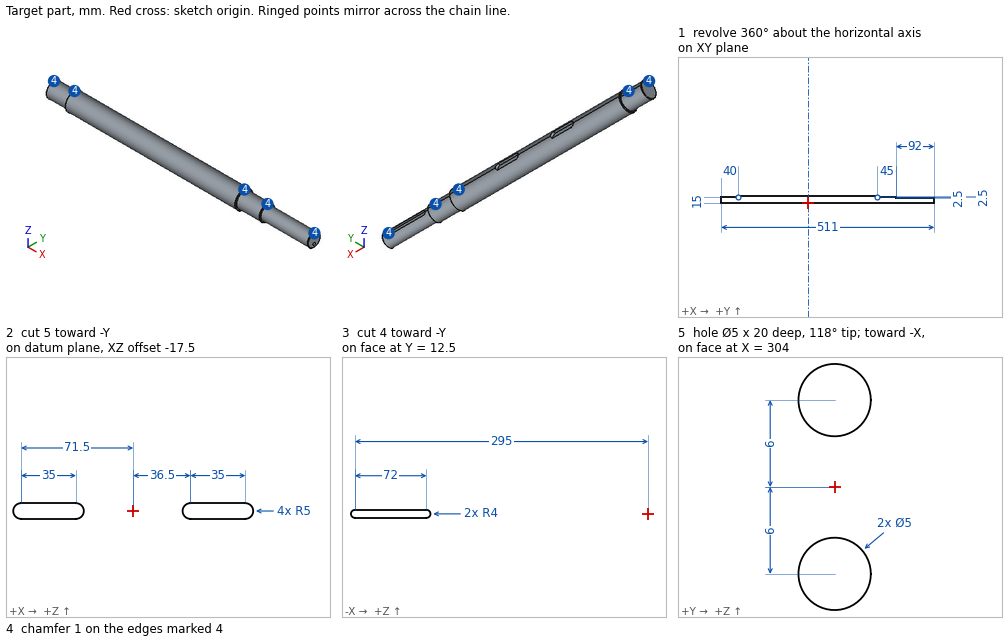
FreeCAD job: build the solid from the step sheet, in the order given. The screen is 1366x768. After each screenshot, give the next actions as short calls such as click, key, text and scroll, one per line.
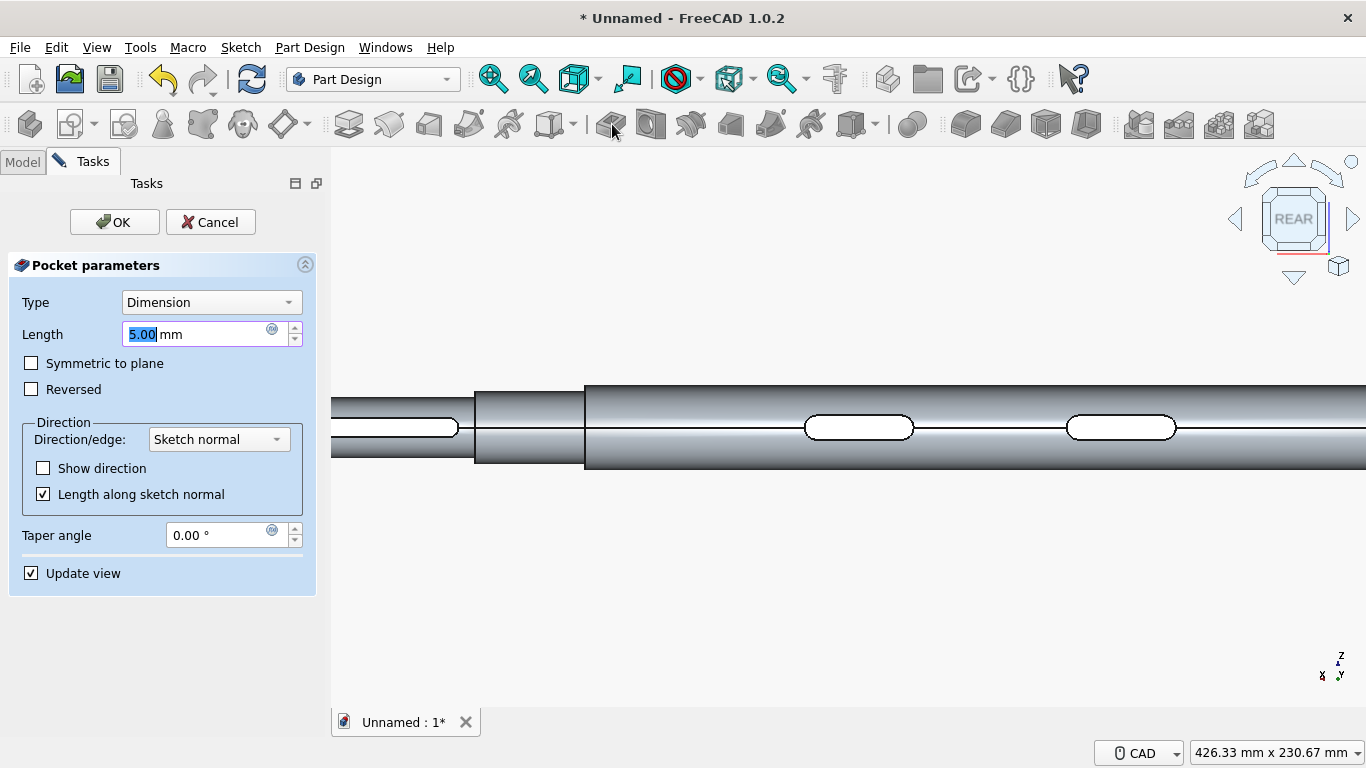
text(4)
key(Tab)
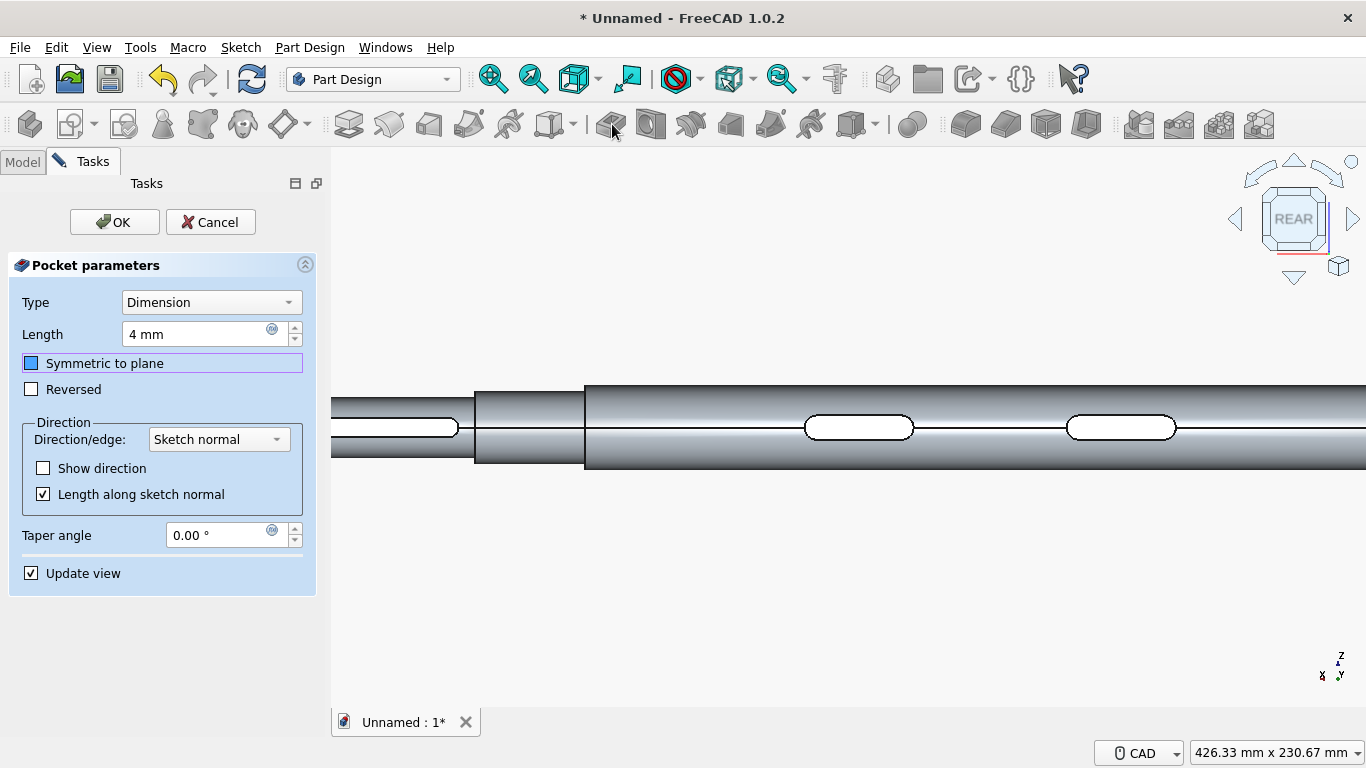
click(115, 222)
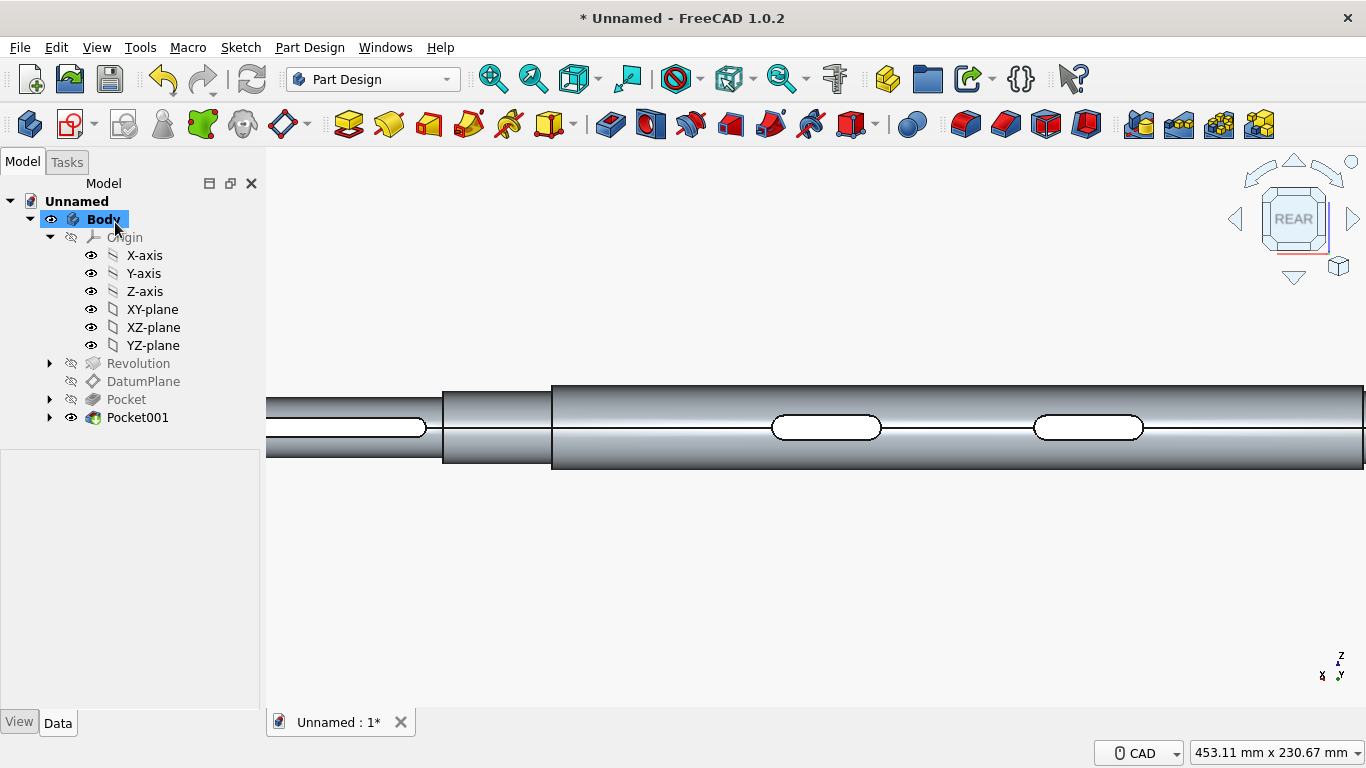
click(494, 80)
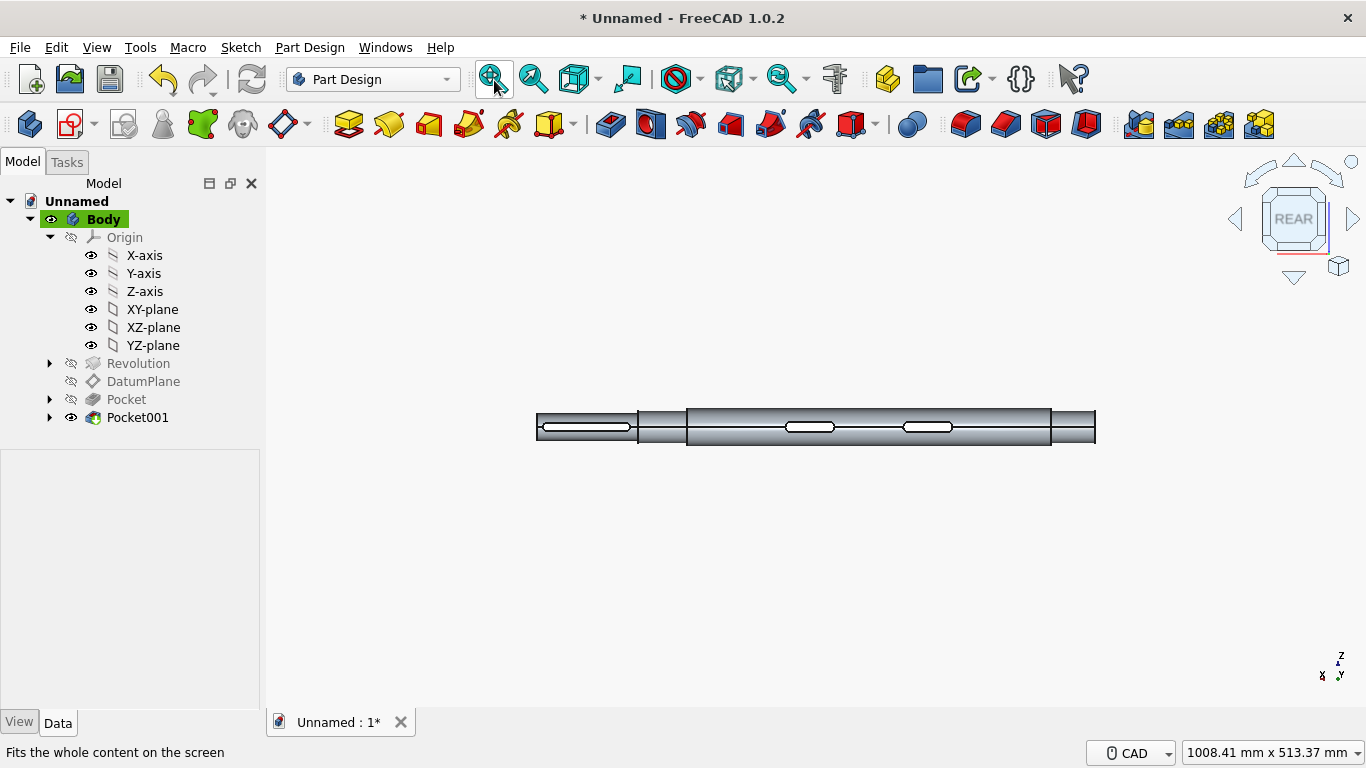
click(1095, 416)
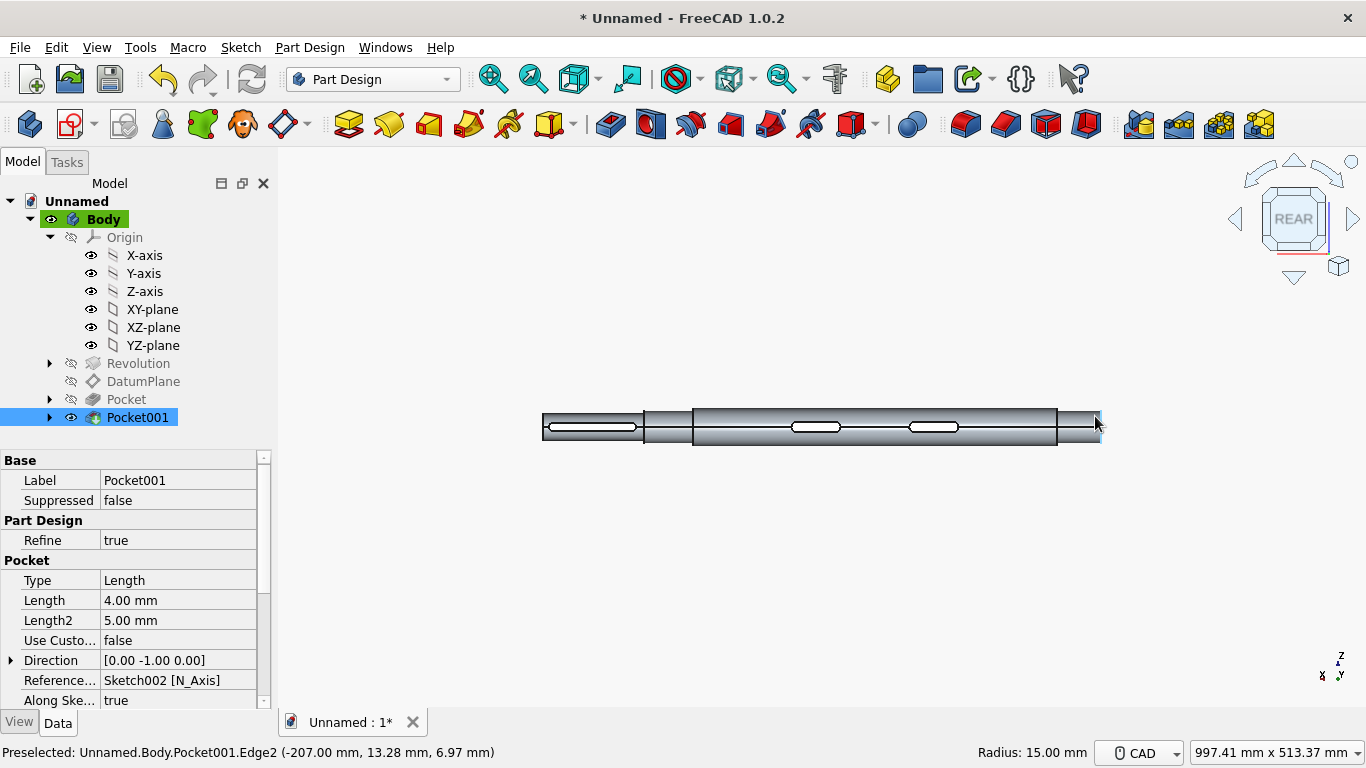
click(1057, 415, ctrl)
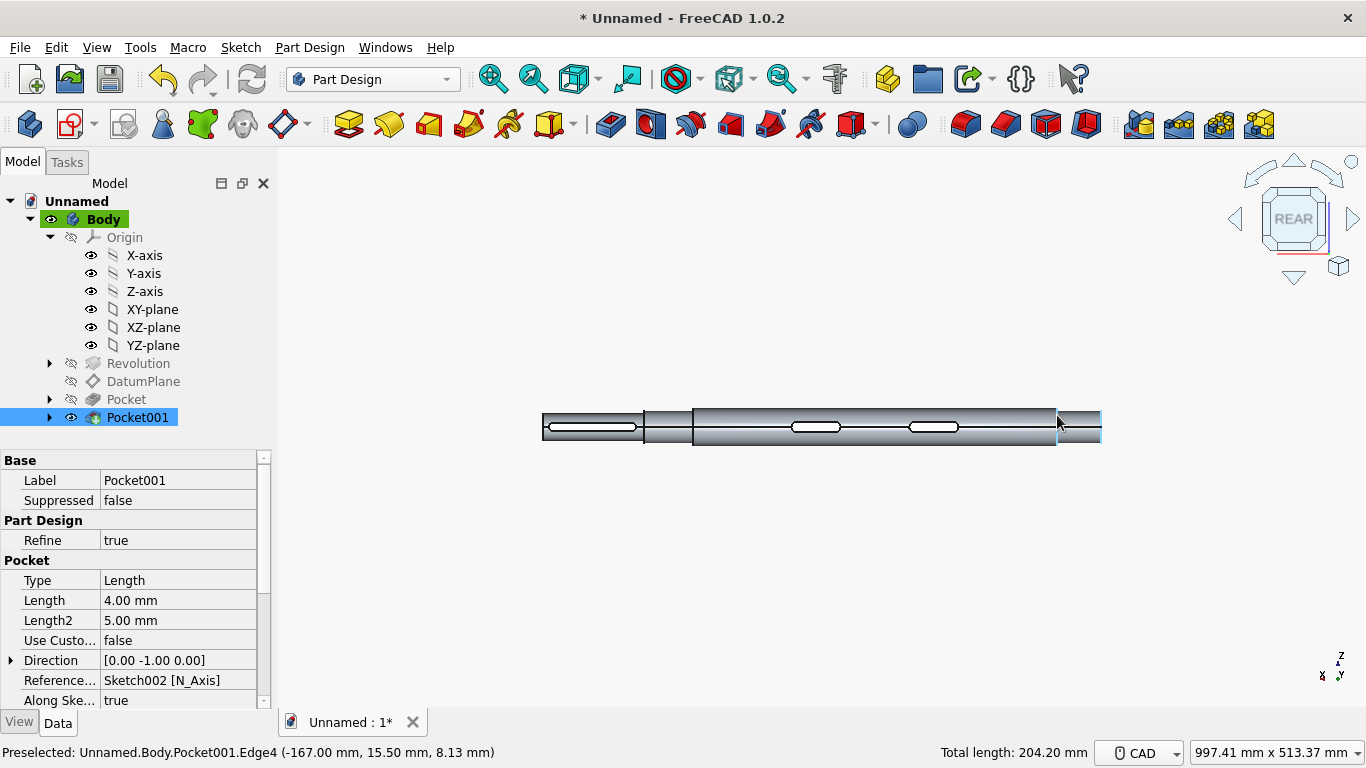
click(693, 415, ctrl)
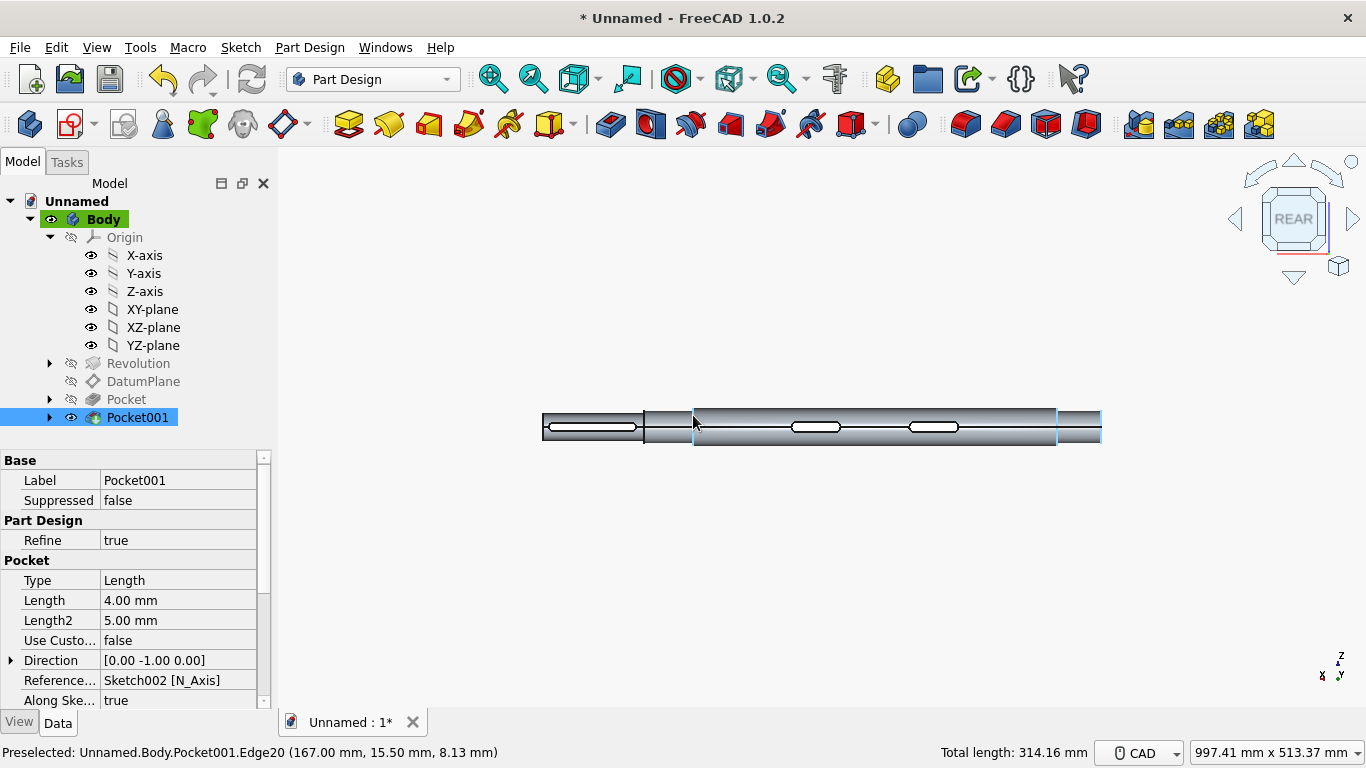
click(644, 416, ctrl)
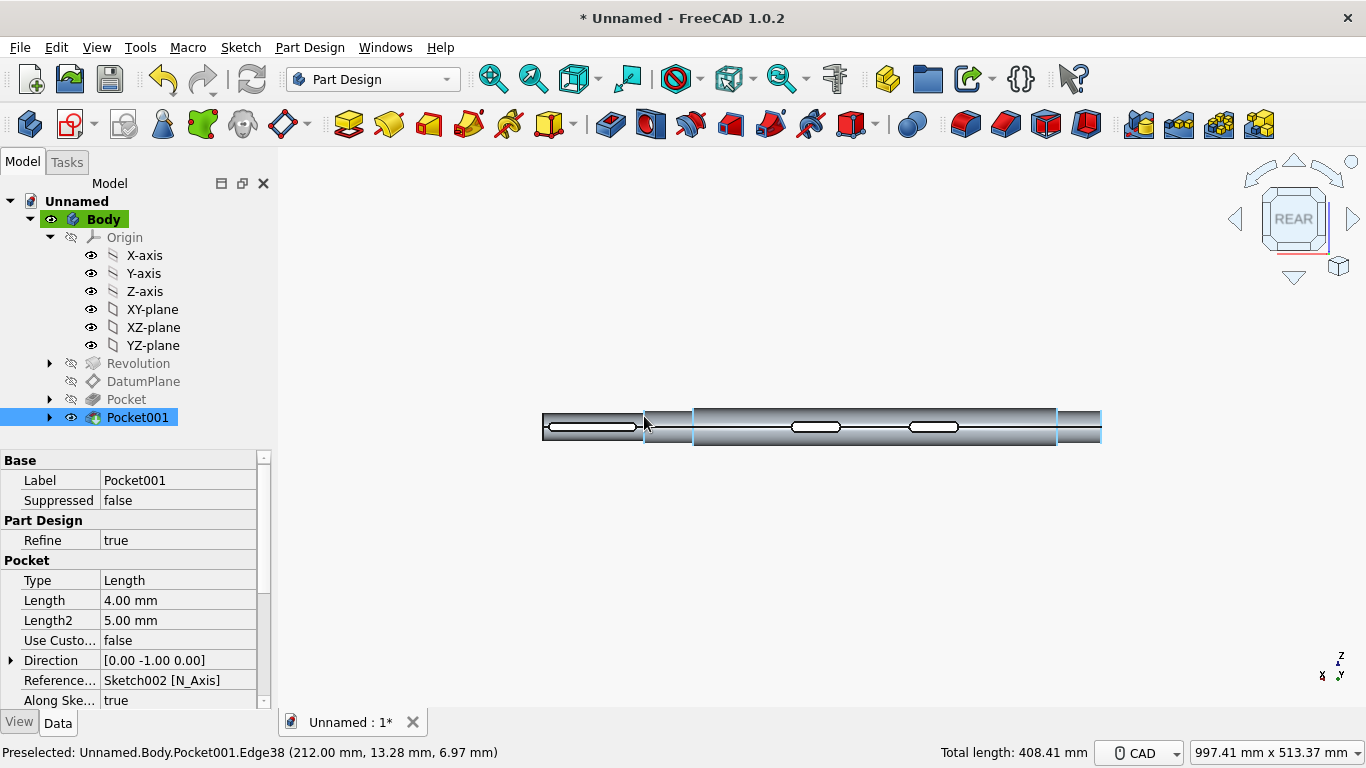
click(543, 418, ctrl)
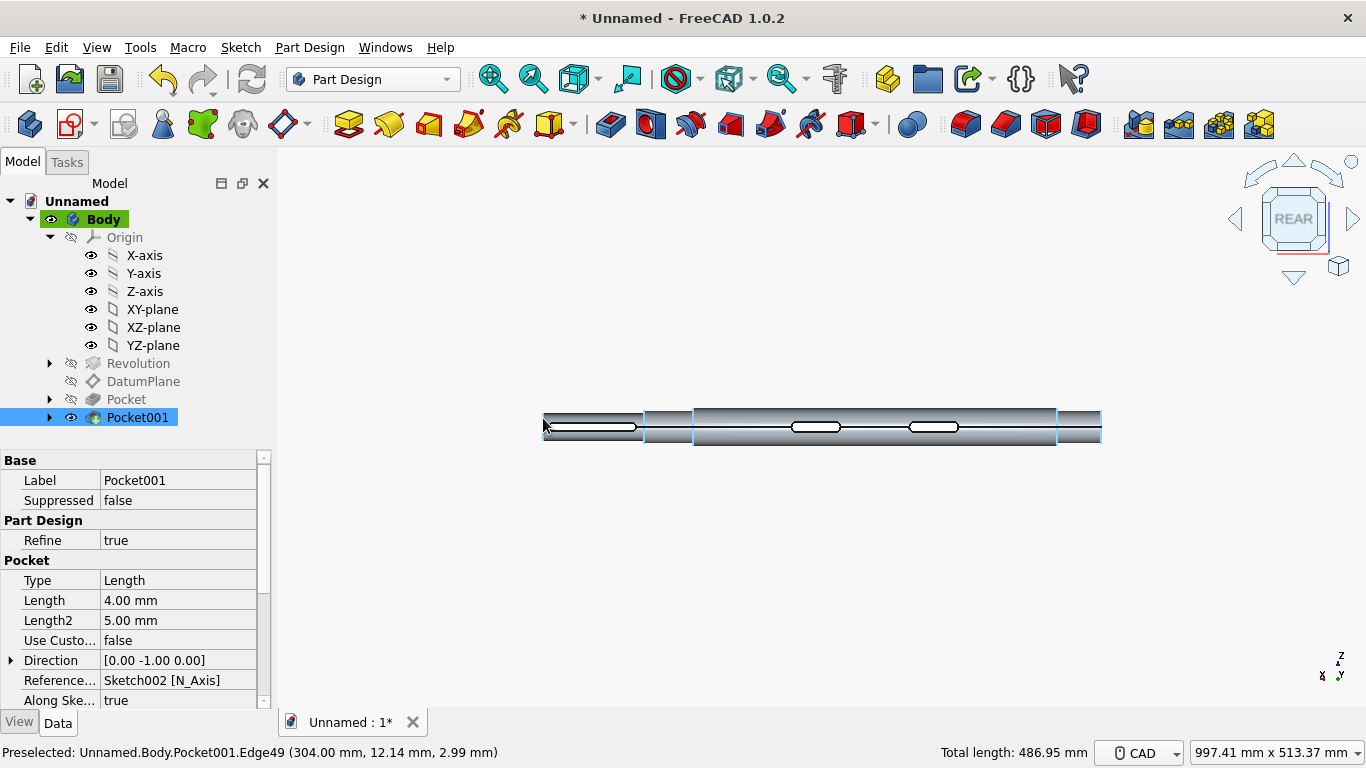
click(1006, 124)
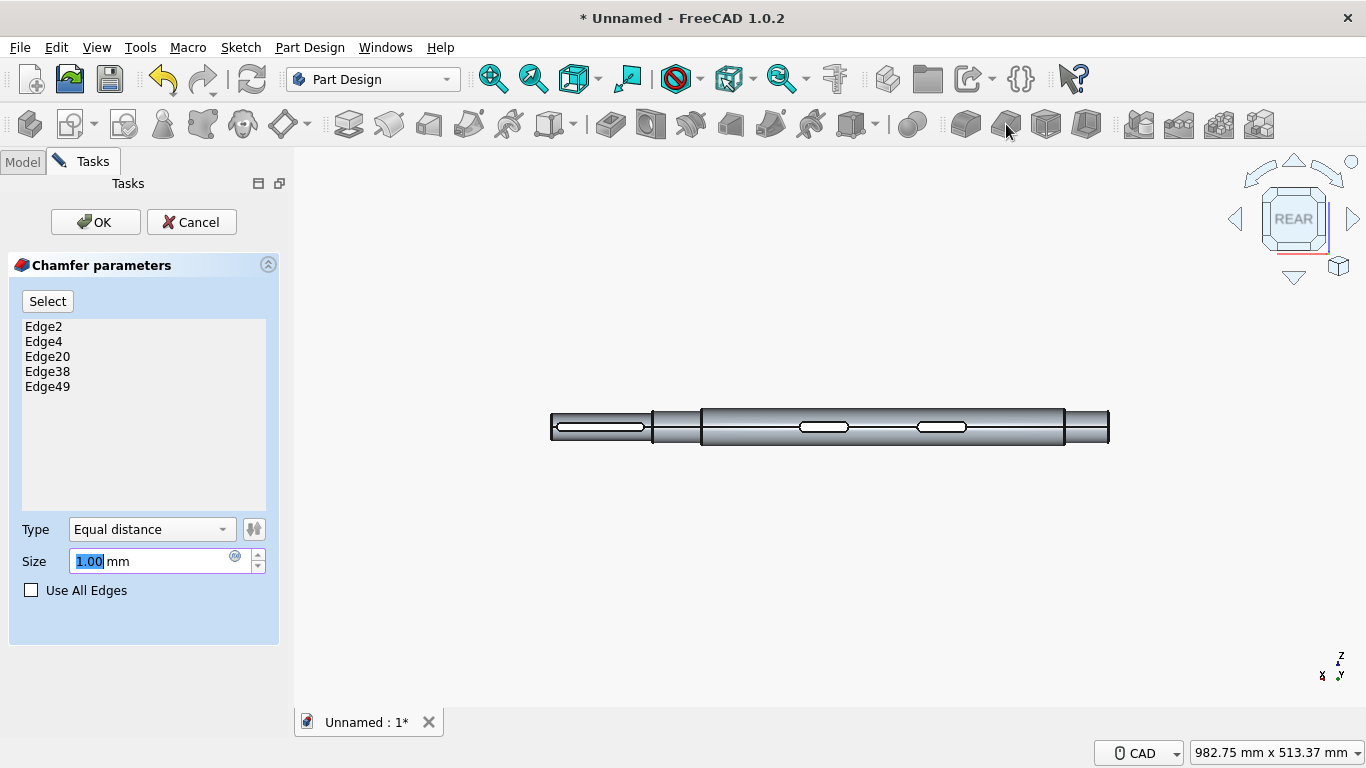
text(1)
key(Tab)